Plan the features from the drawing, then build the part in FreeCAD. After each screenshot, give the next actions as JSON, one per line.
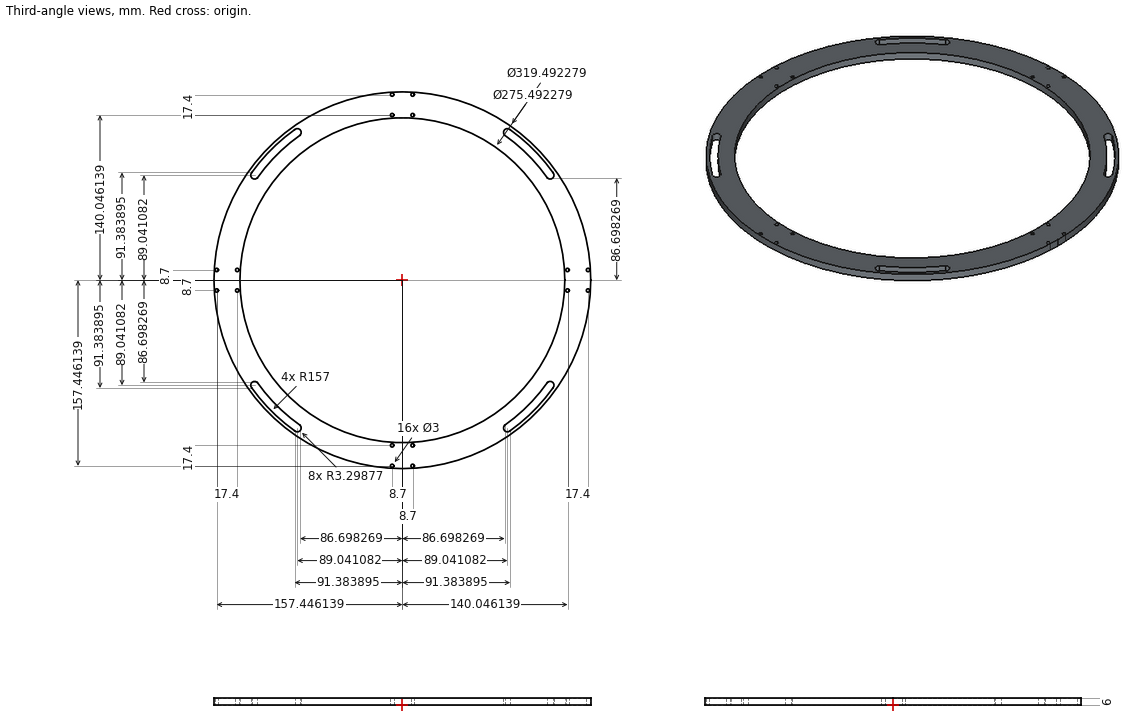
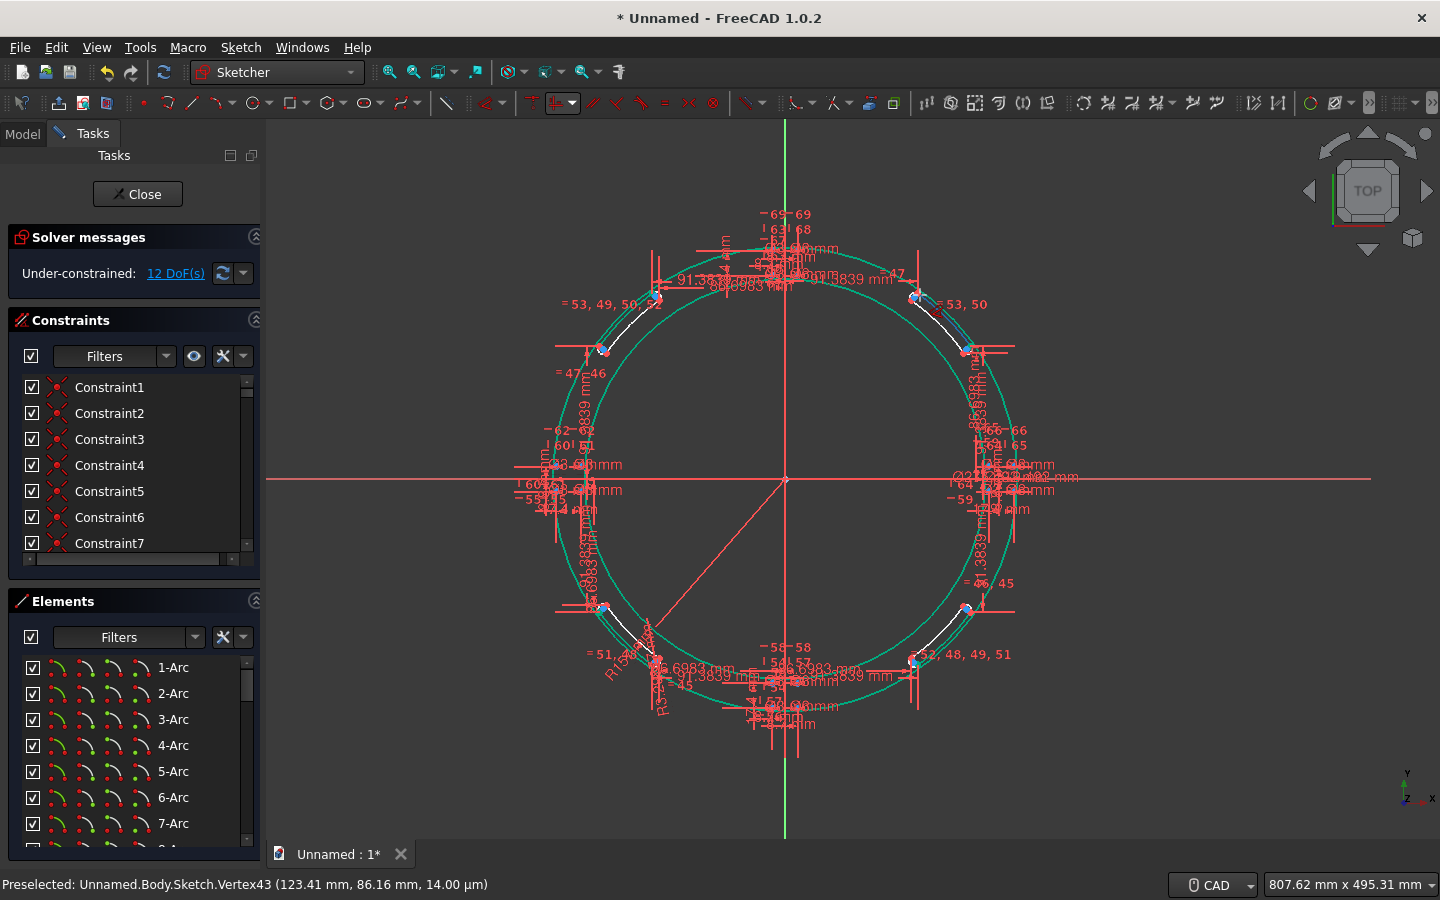
{"action": "scroll", "coordinate": [656, 661], "scroll_direction": "up", "scroll_amount": 5}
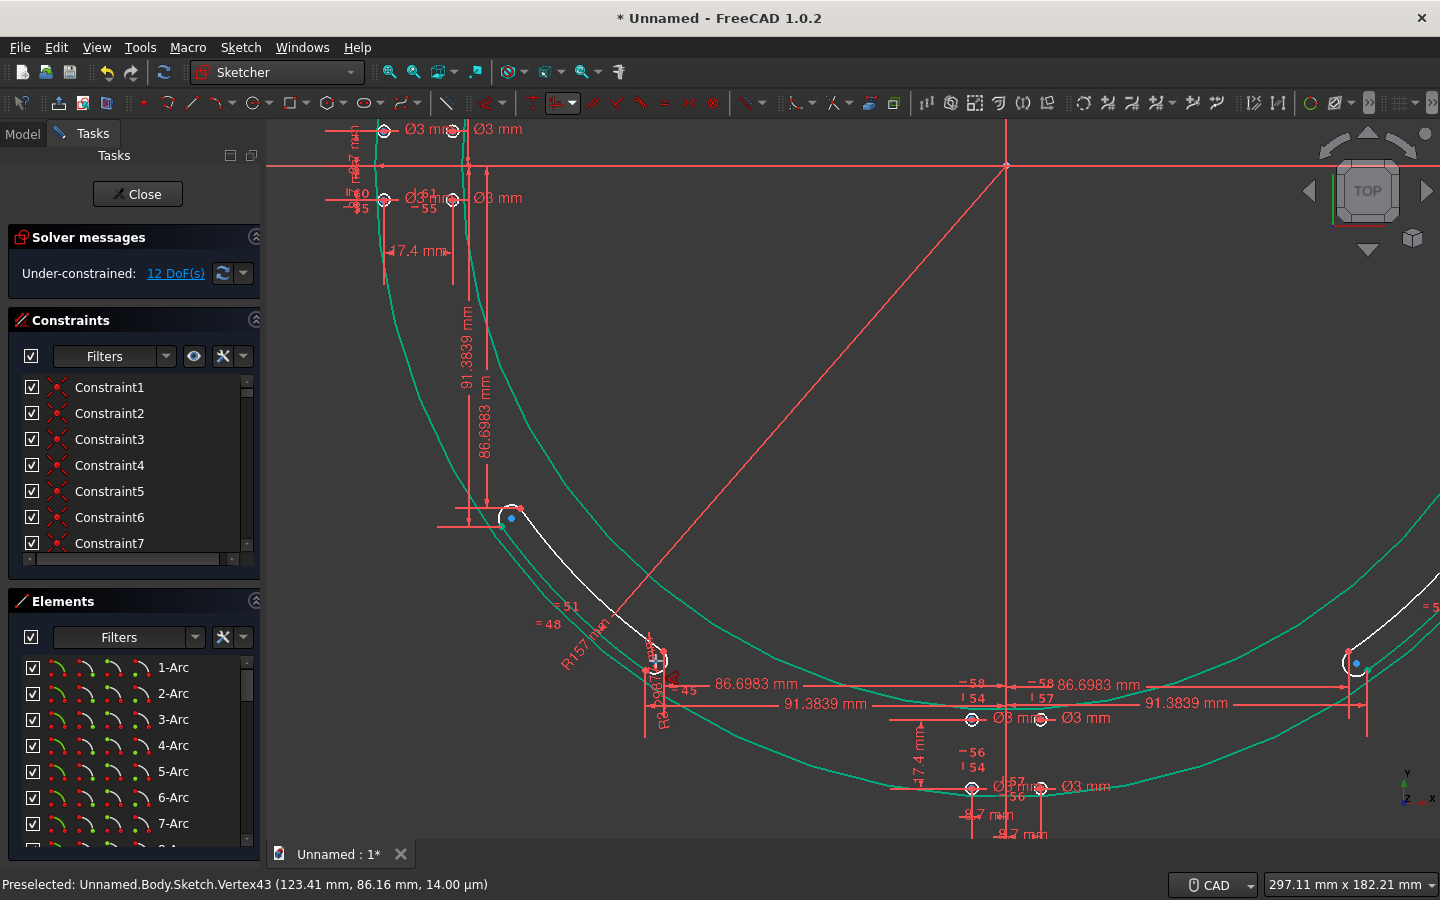
{"action": "left_click", "coordinate": [654, 661]}
{"action": "left_click", "coordinate": [749, 719]}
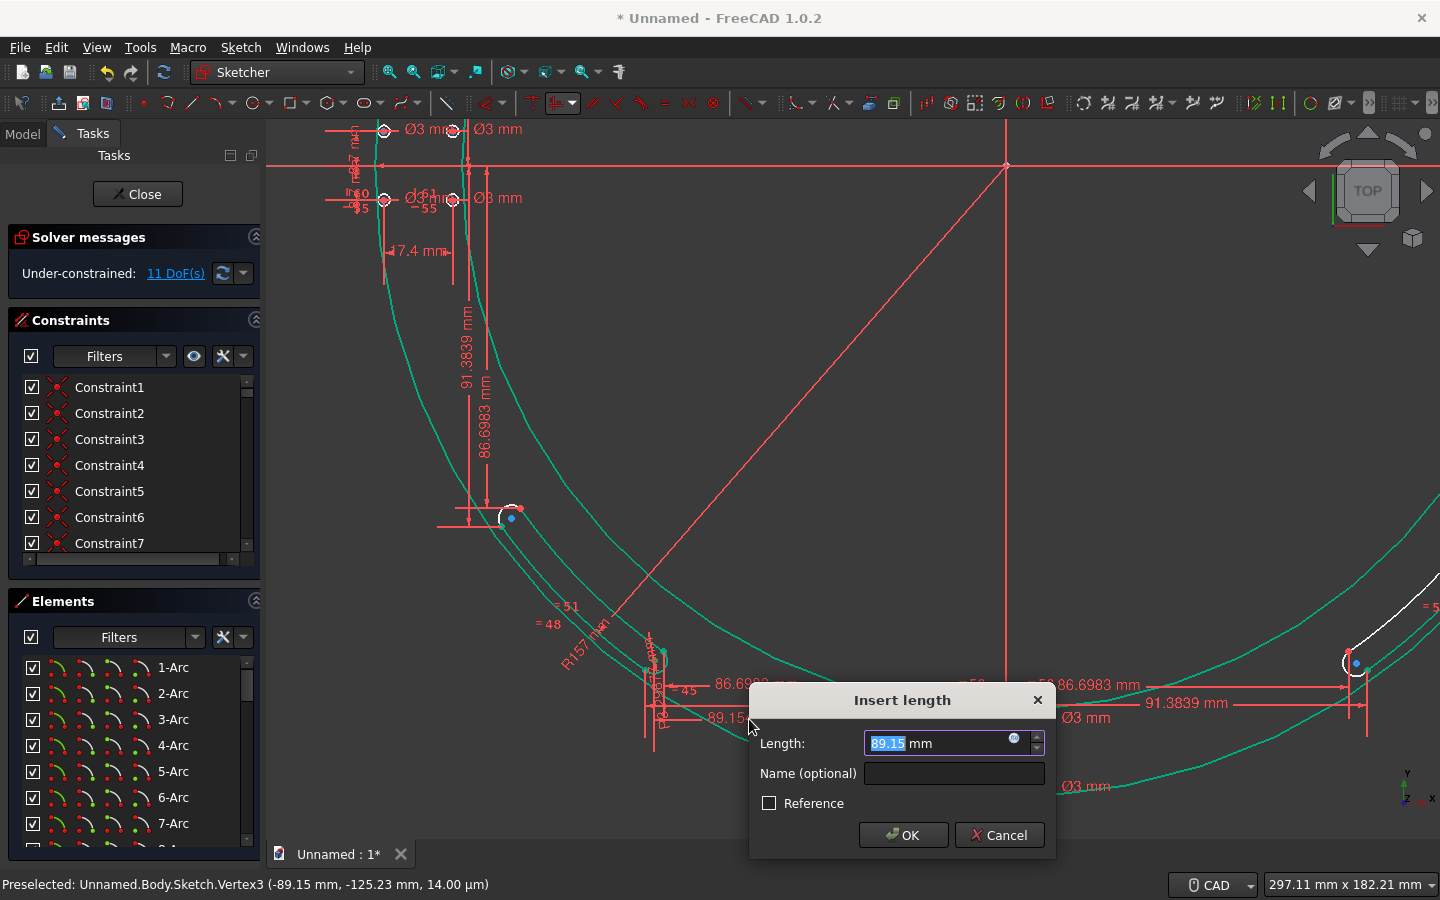
{"action": "type", "text": "89.041082"}
{"action": "key", "text": "Return"}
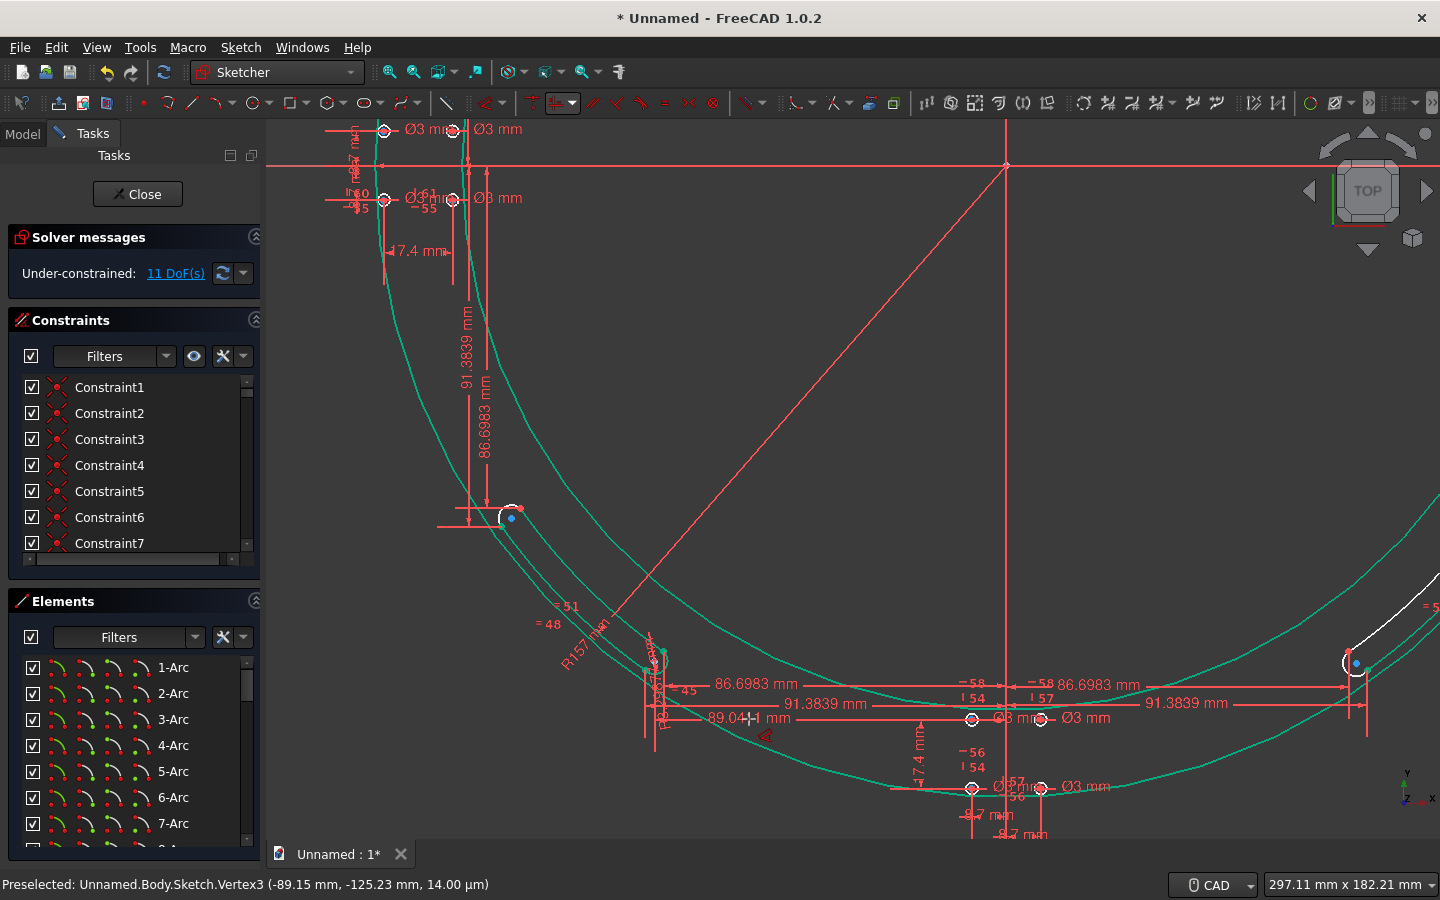
{"action": "left_click", "coordinate": [512, 518]}
{"action": "left_click", "coordinate": [478, 465]}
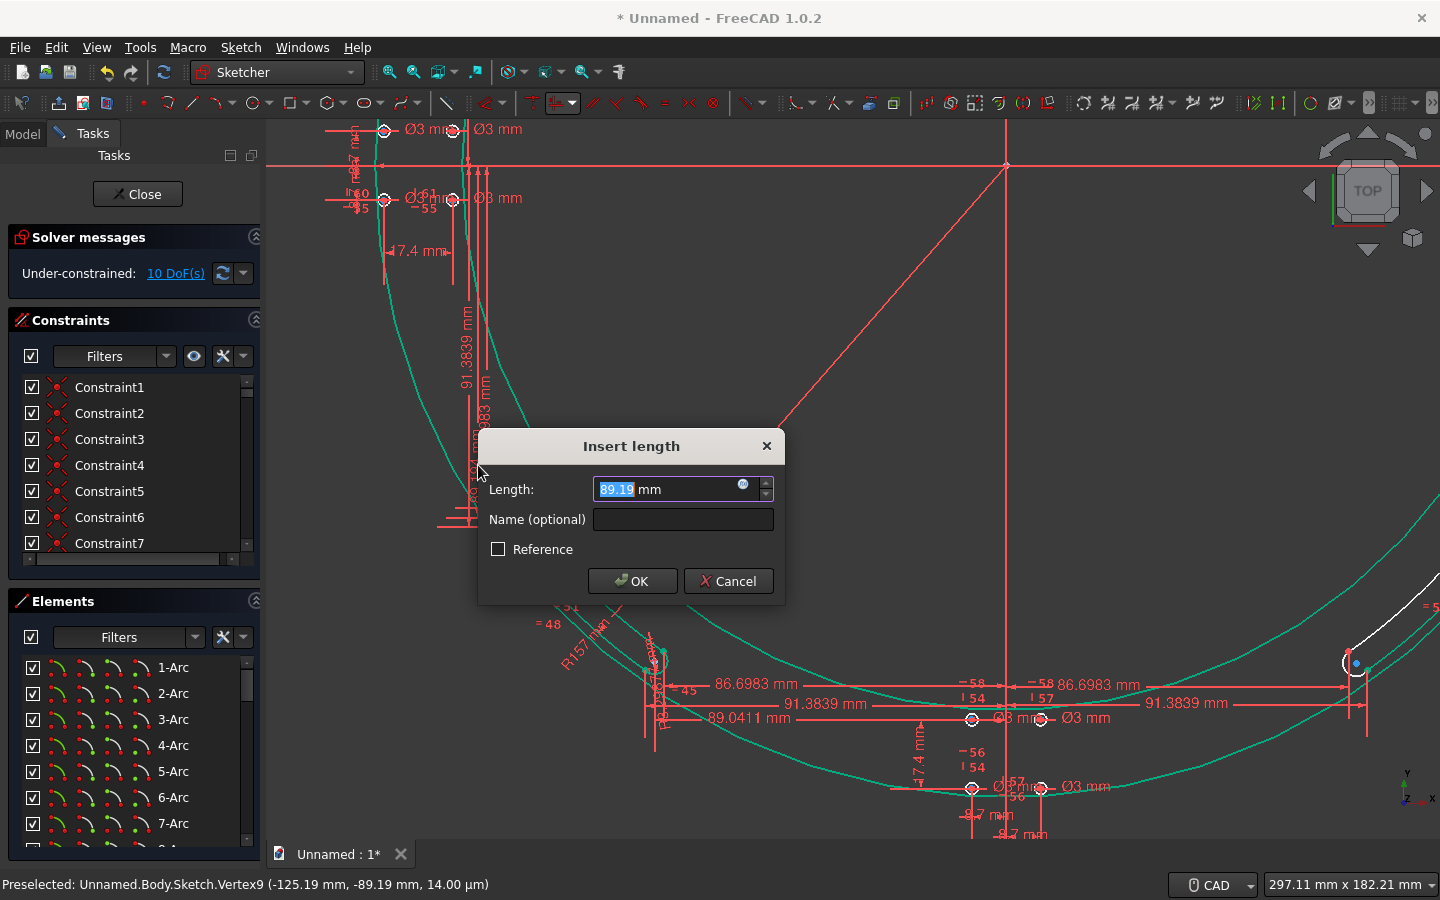
{"action": "type", "text": "89.041082"}
{"action": "key", "text": "Return"}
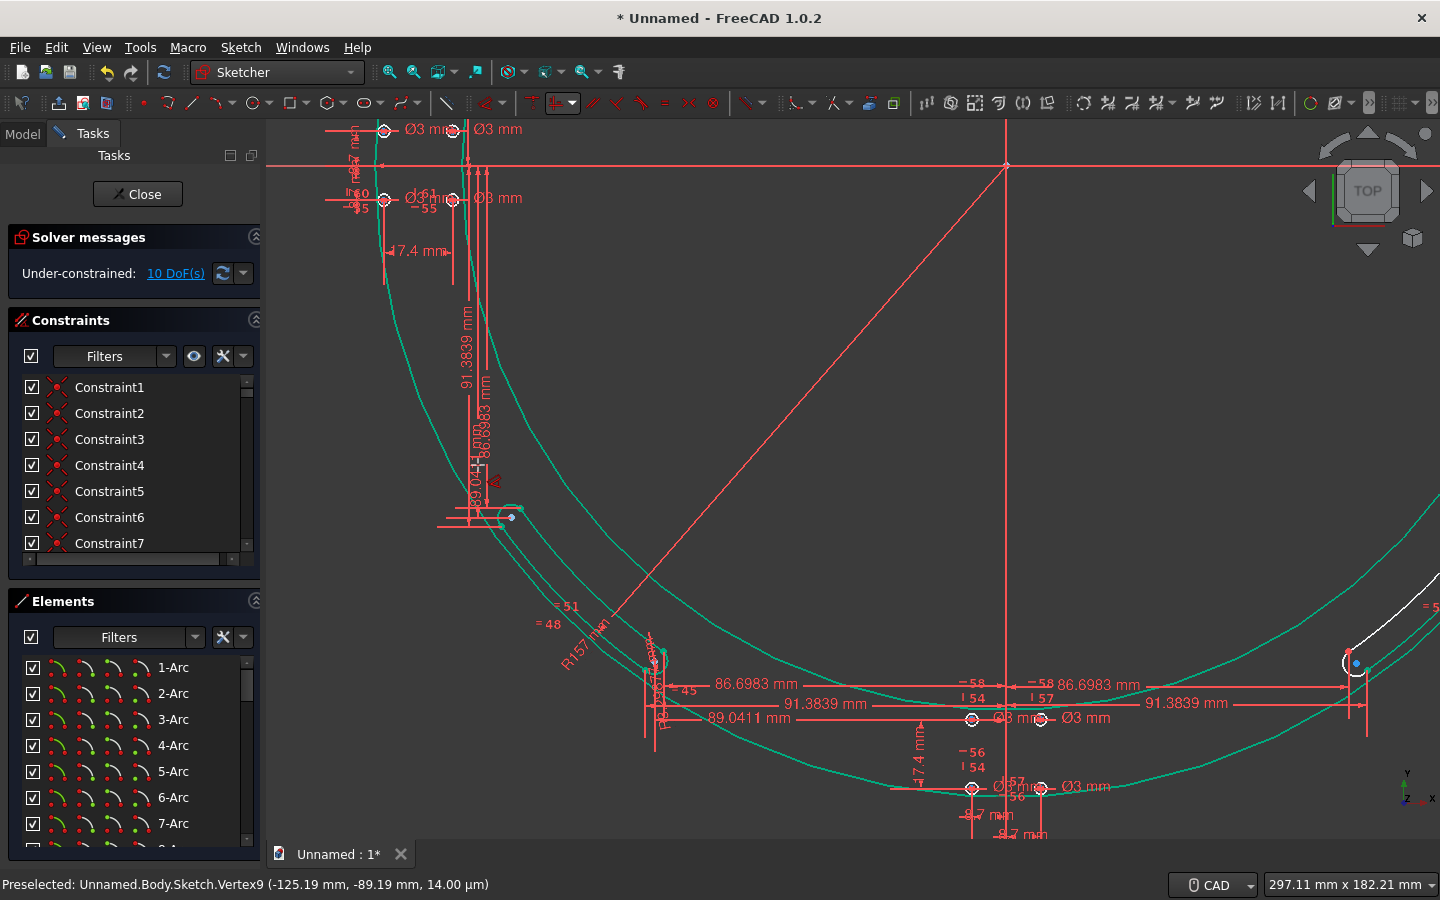
{"action": "scroll", "coordinate": [655, 661], "scroll_direction": "down", "scroll_amount": 5}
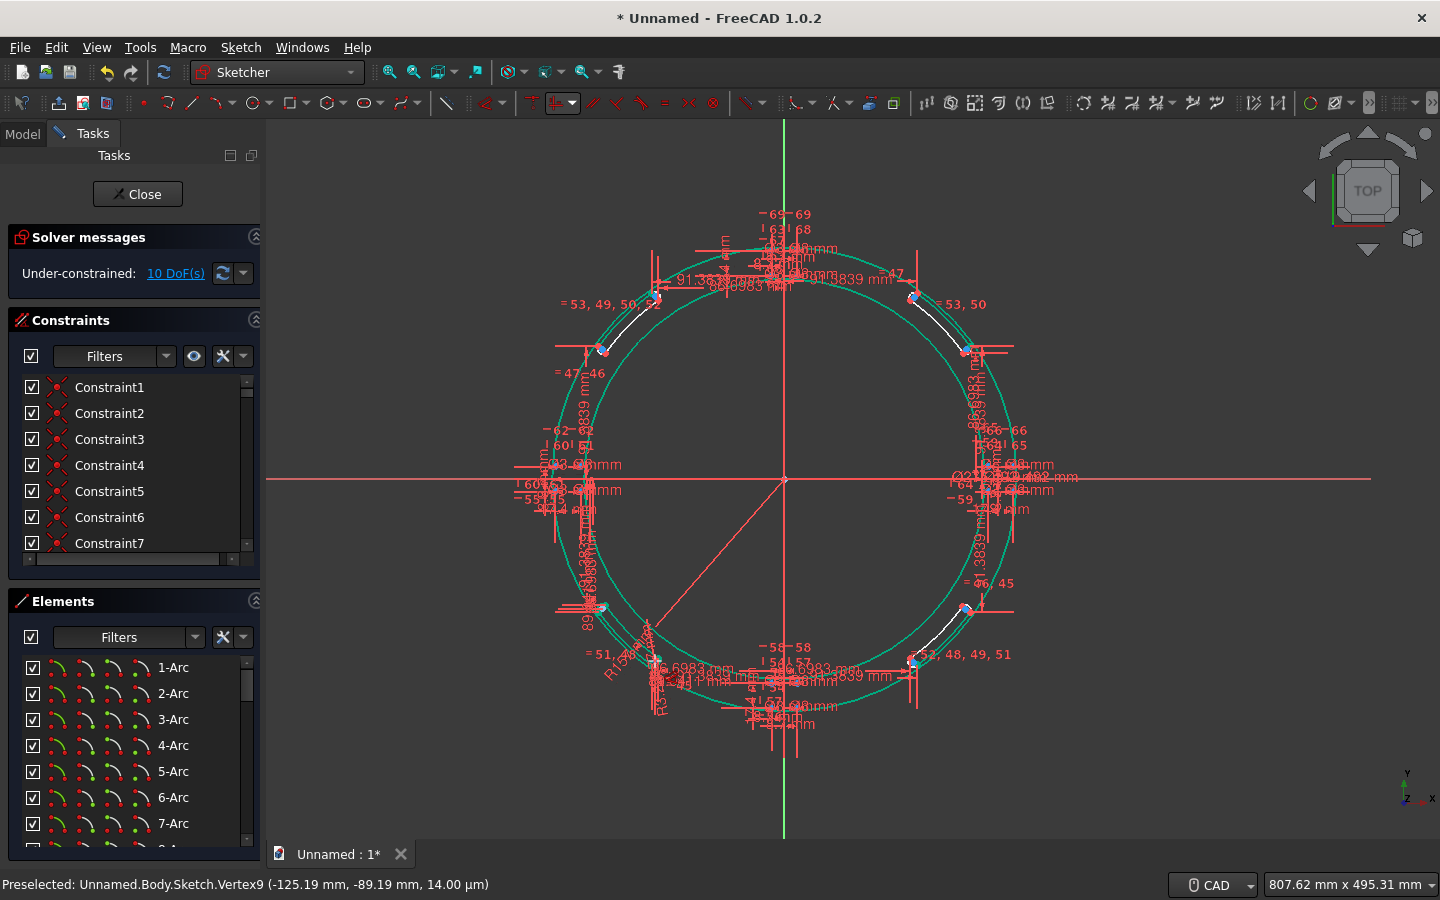
{"action": "scroll", "coordinate": [966, 610], "scroll_direction": "up", "scroll_amount": 5}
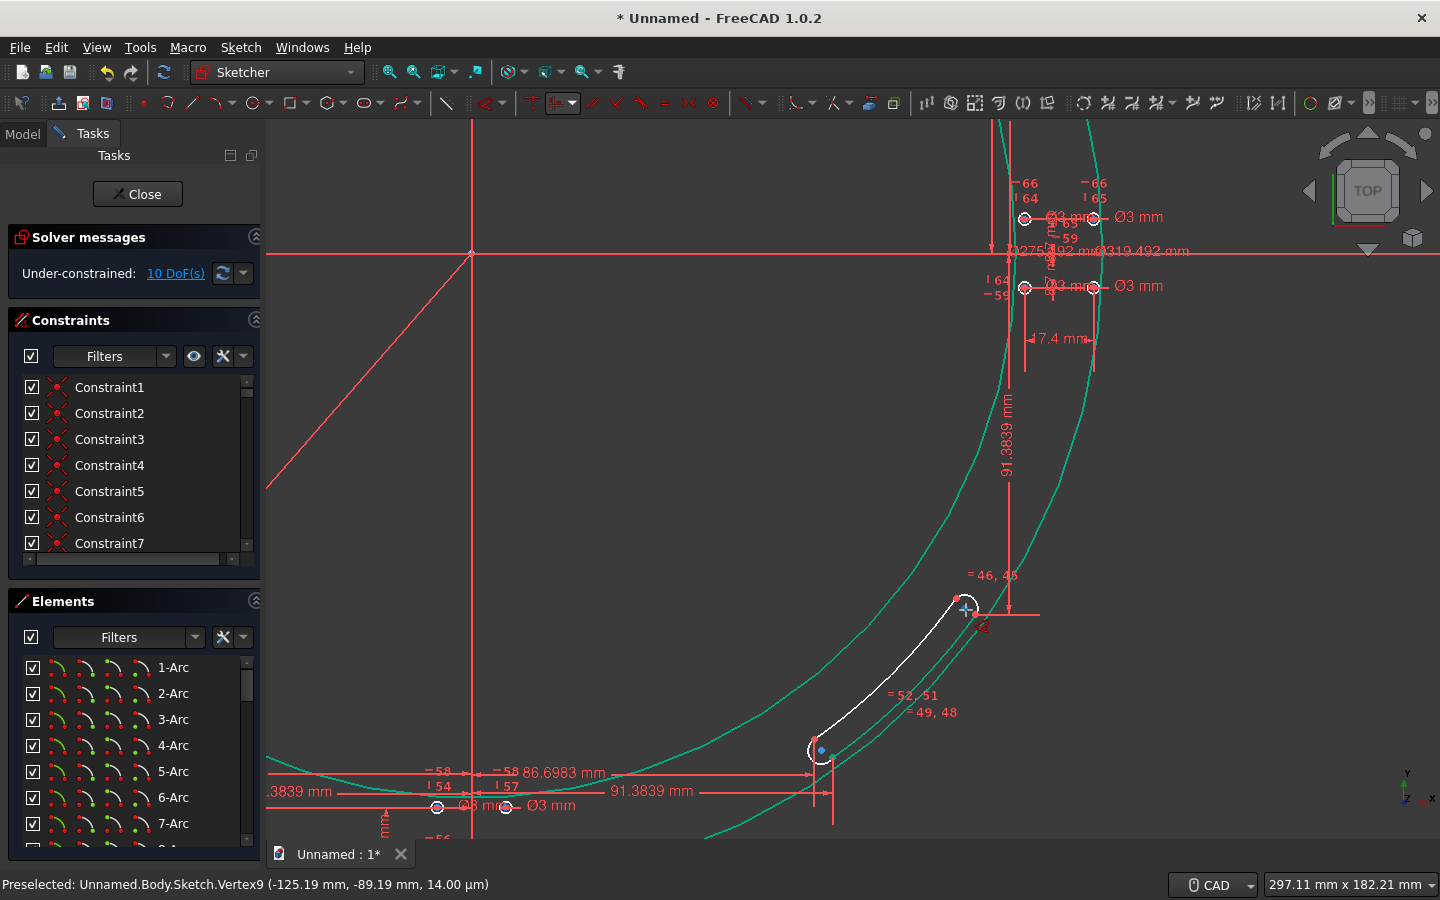
{"action": "left_click", "coordinate": [965, 608]}
{"action": "left_click", "coordinate": [999, 512]}